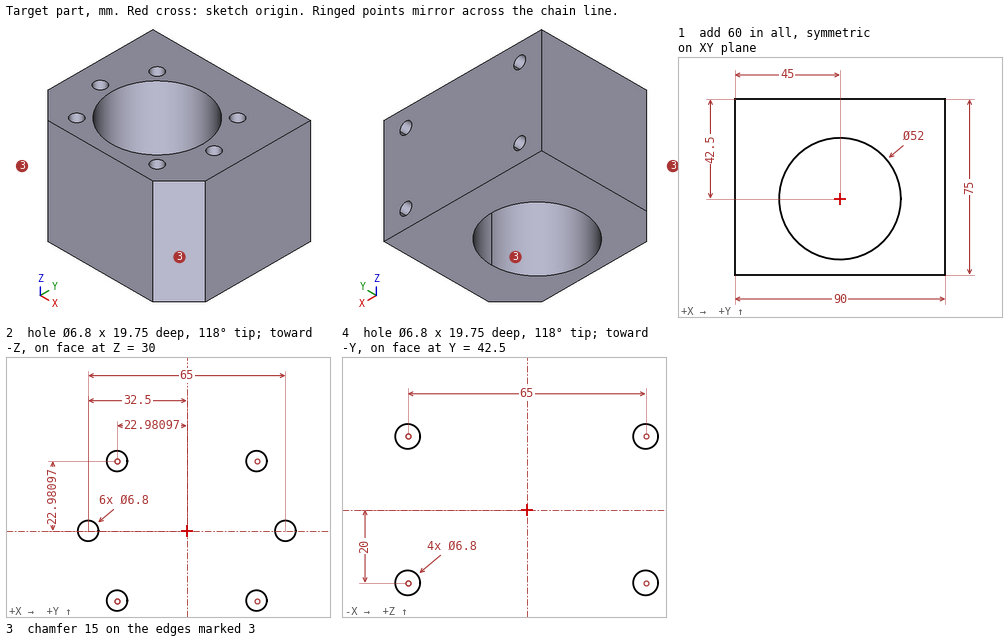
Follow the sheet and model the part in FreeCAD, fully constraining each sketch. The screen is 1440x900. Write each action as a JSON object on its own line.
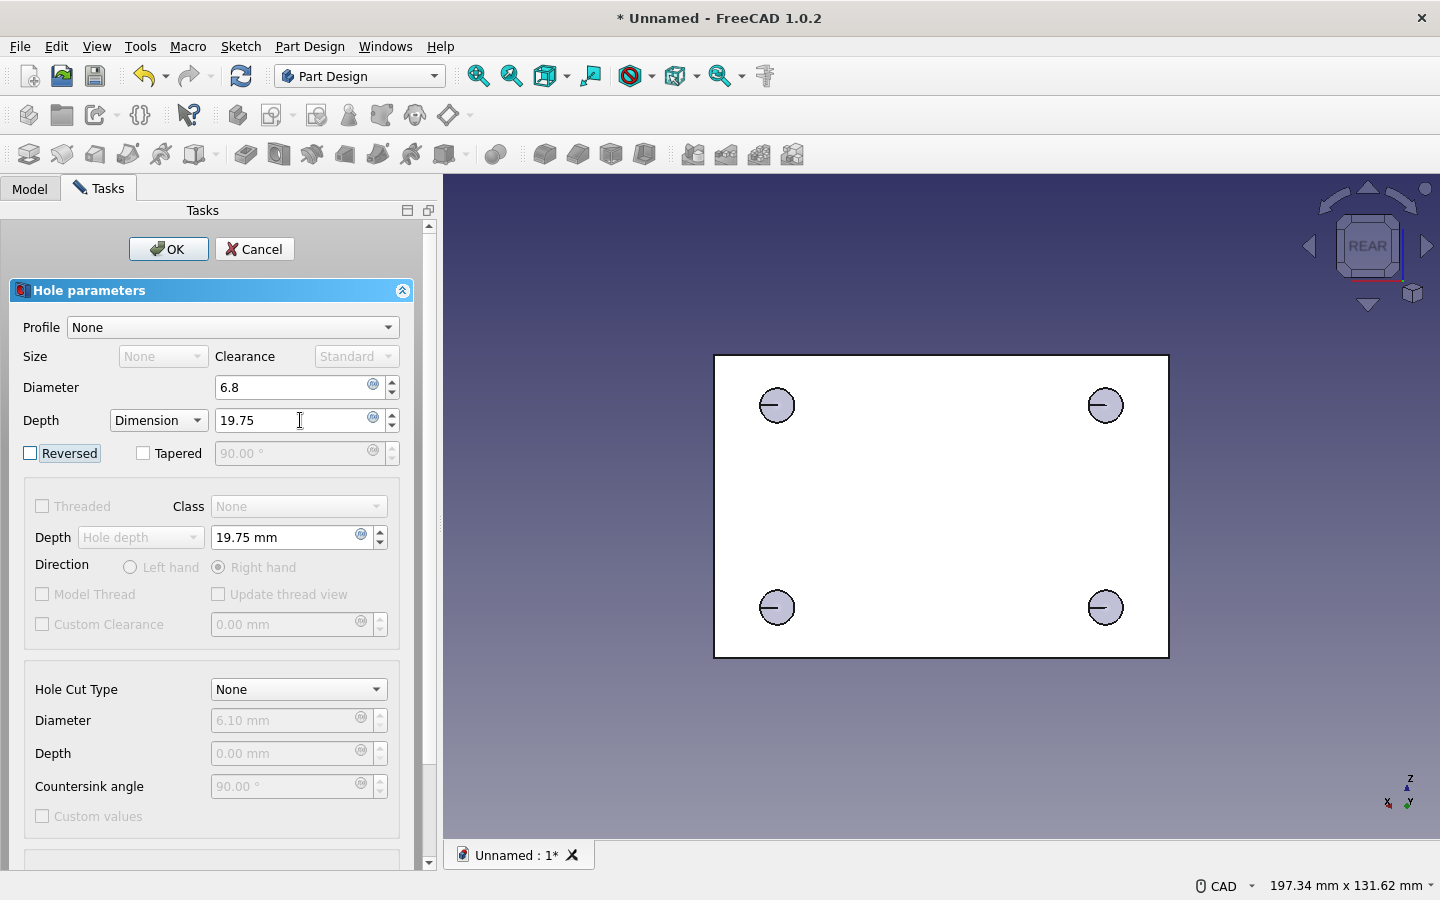
{"action": "left_click", "coordinate": [169, 249]}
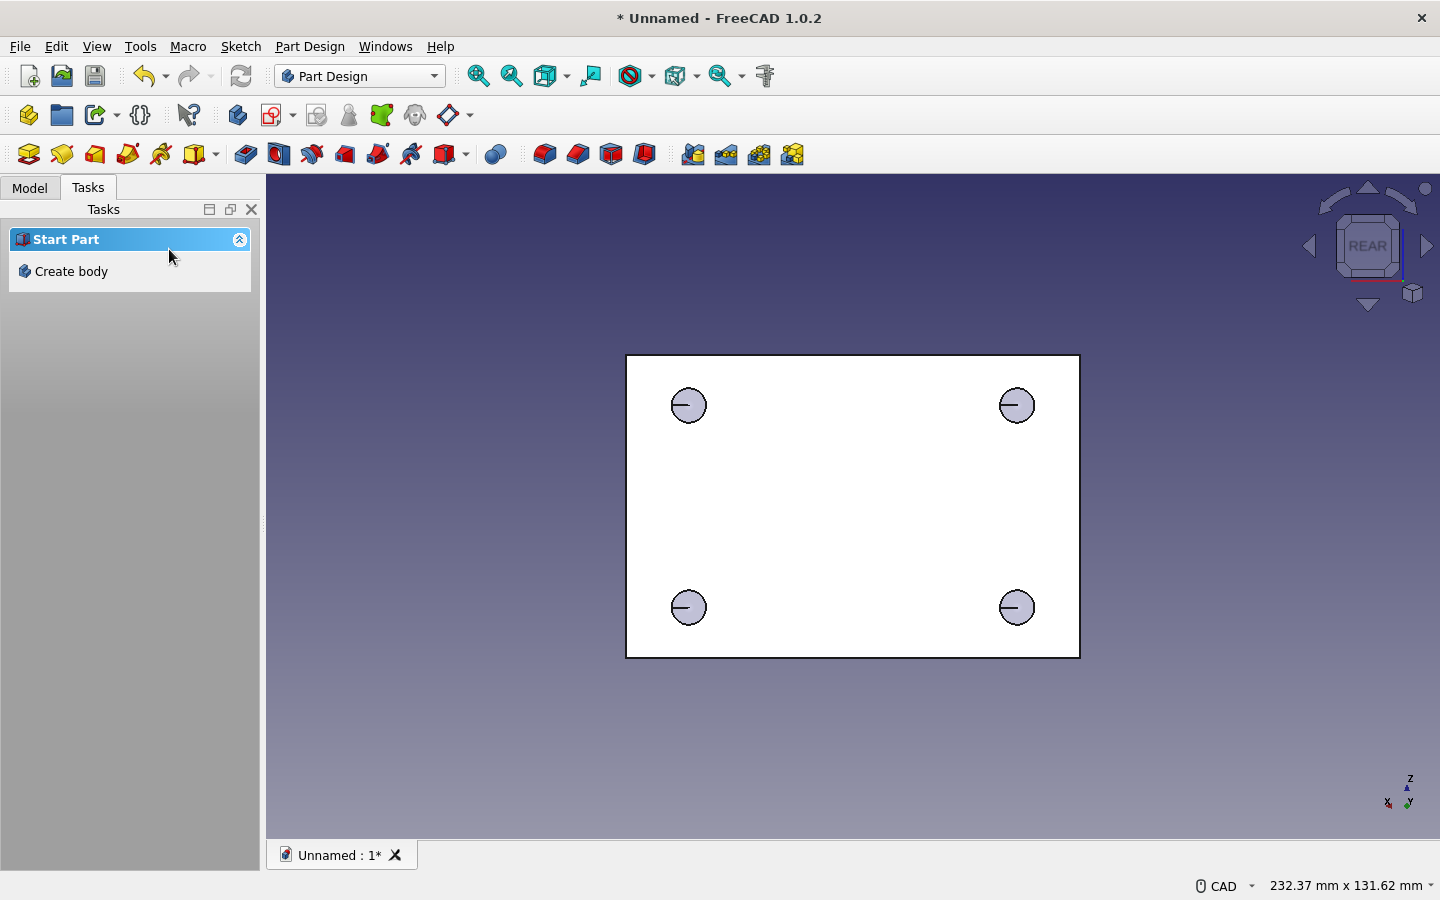
{"action": "key", "text": "0"}